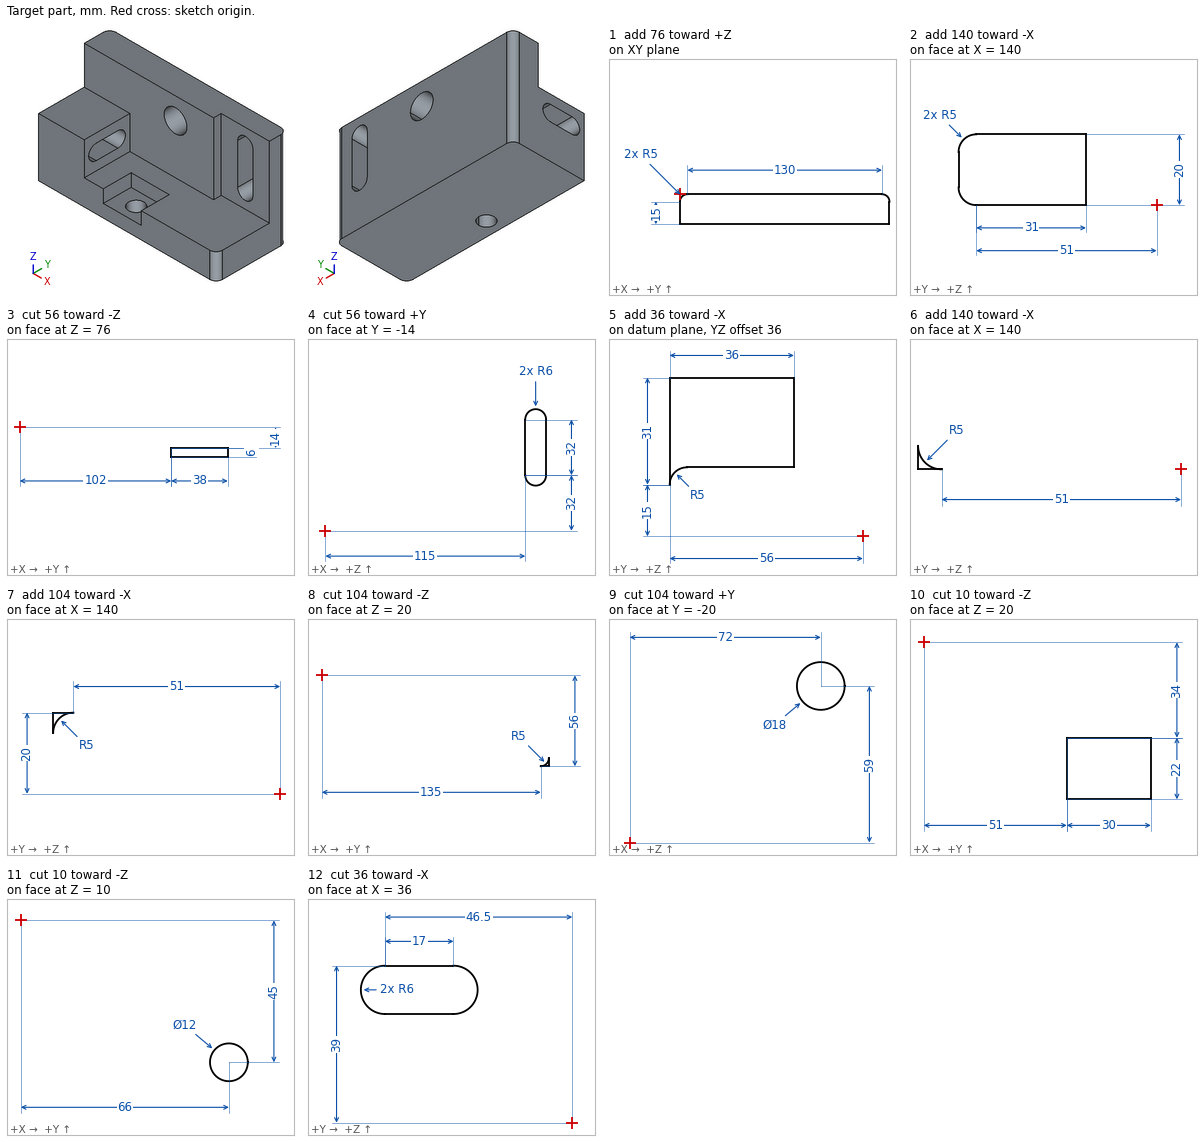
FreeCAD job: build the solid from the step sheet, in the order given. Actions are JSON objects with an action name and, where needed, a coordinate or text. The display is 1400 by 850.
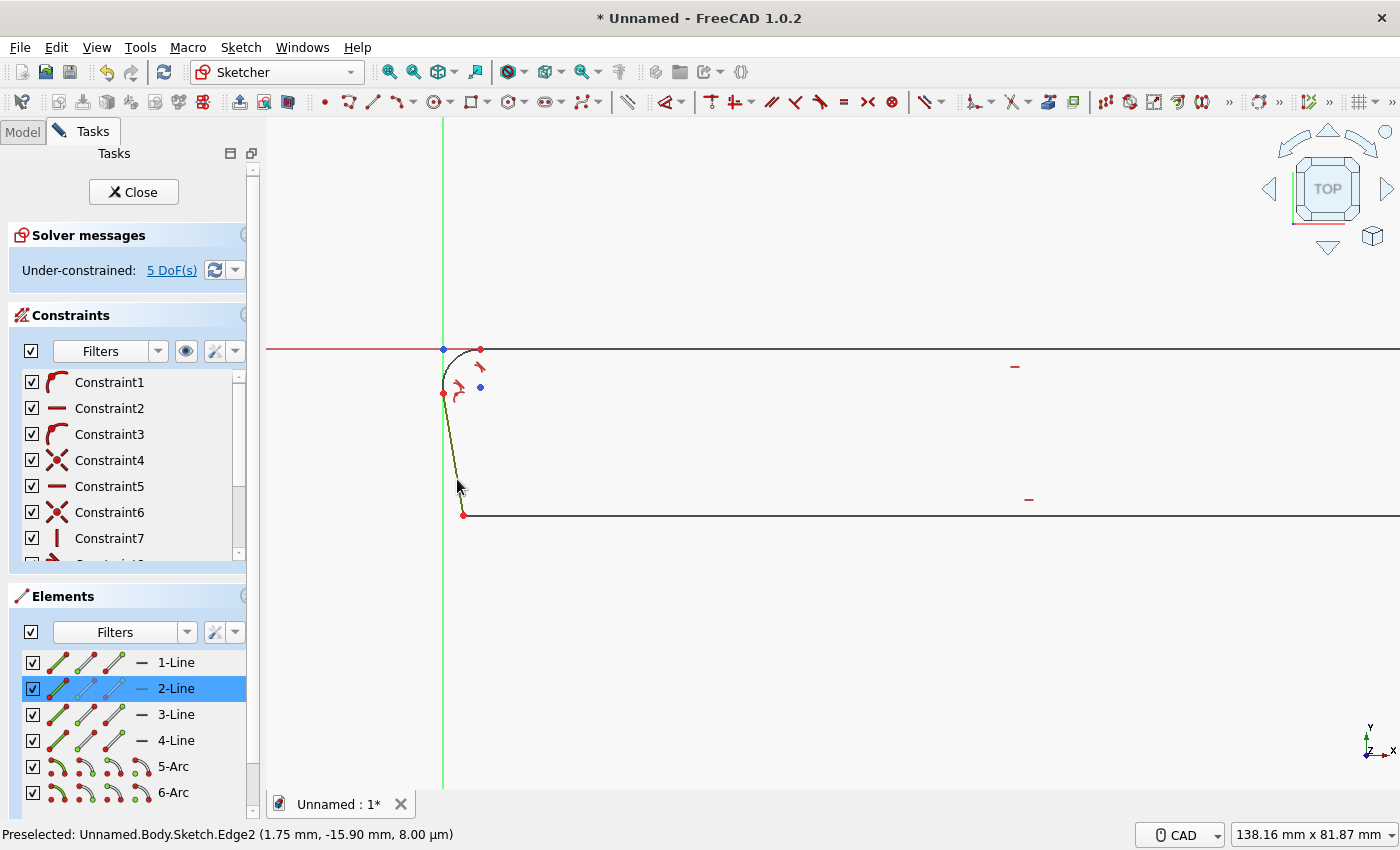
{"action": "key", "text": "v"}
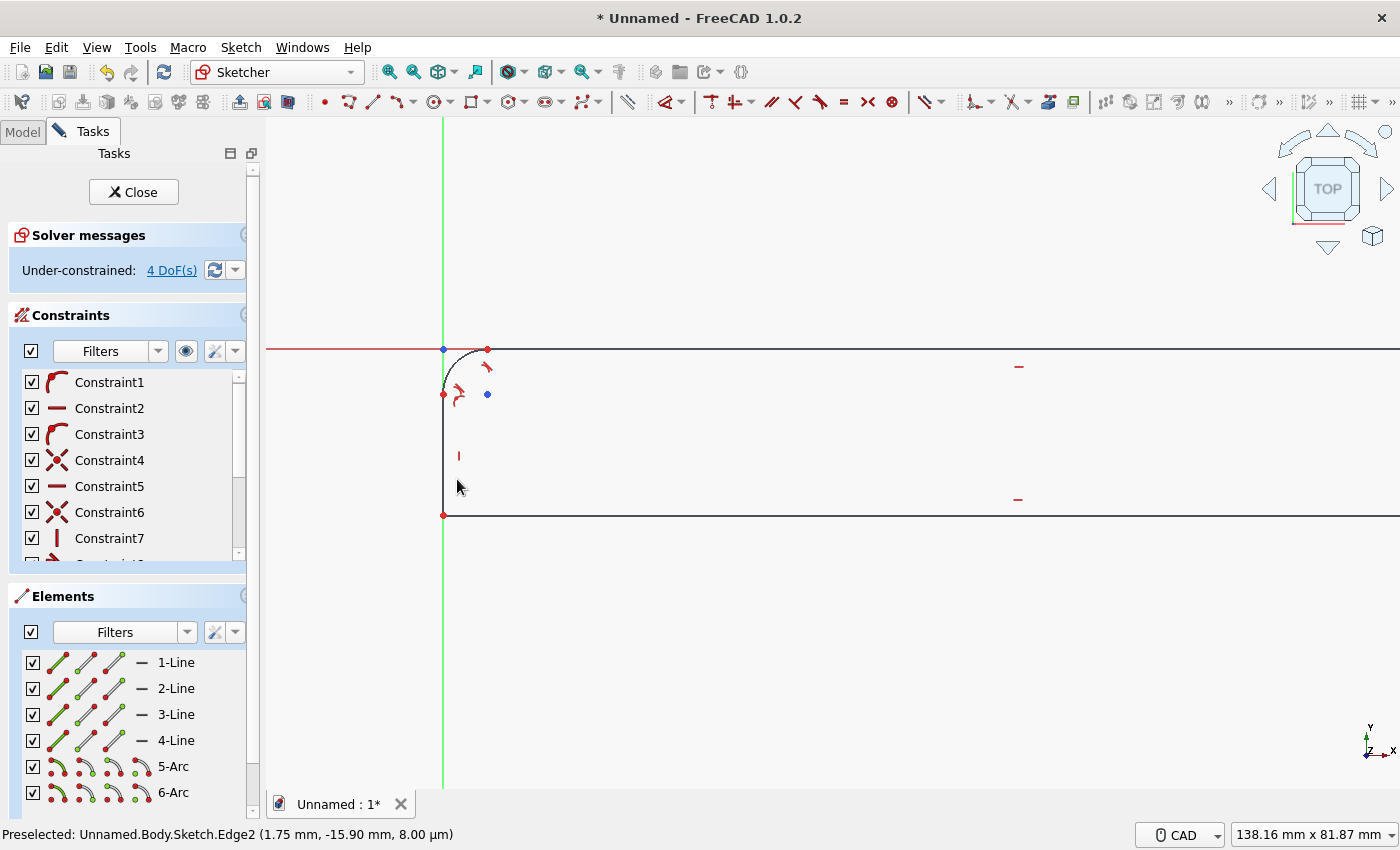
{"action": "left_click", "coordinate": [456, 362]}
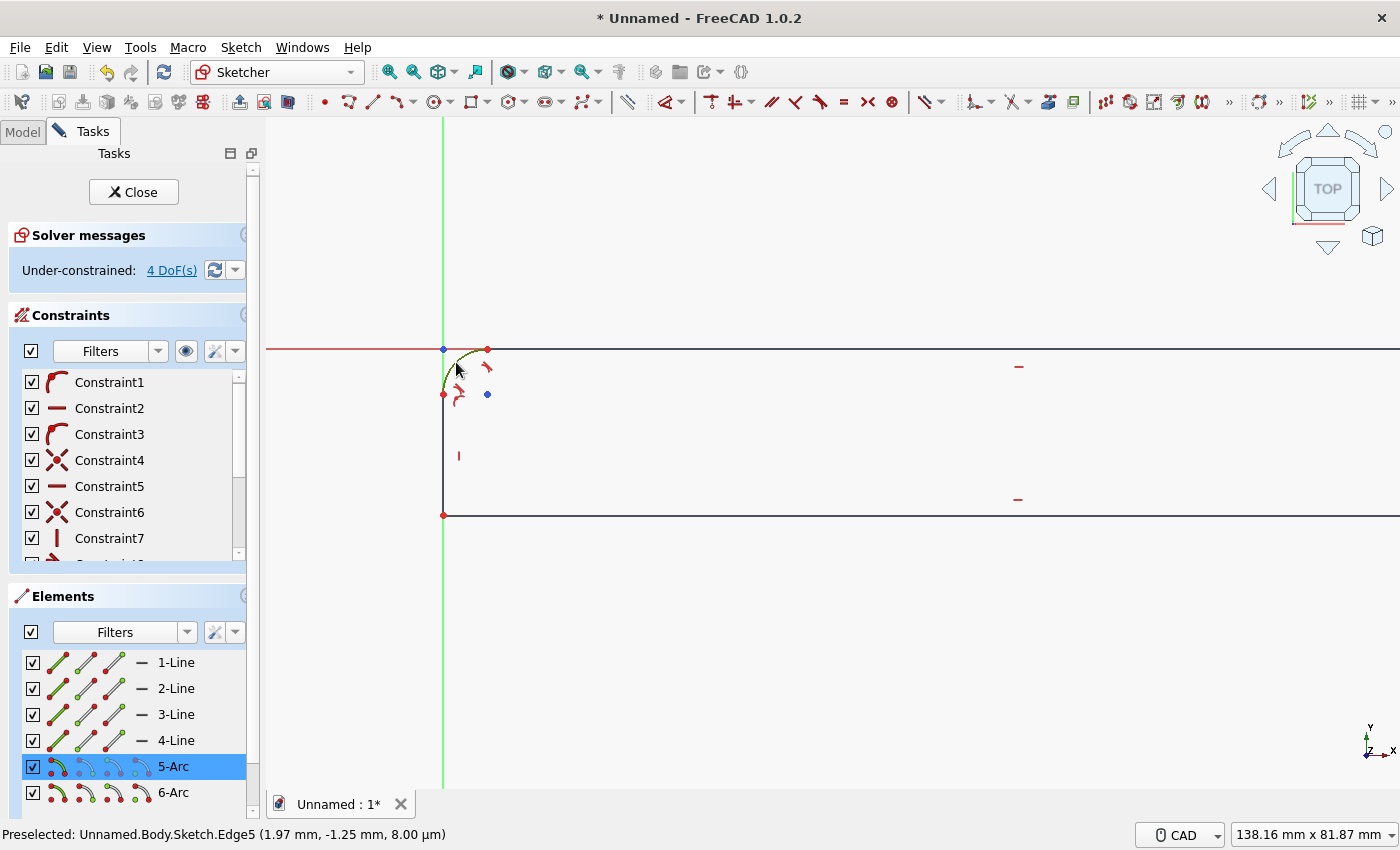
{"action": "scroll", "coordinate": [457, 479], "scroll_direction": "down", "scroll_amount": 3}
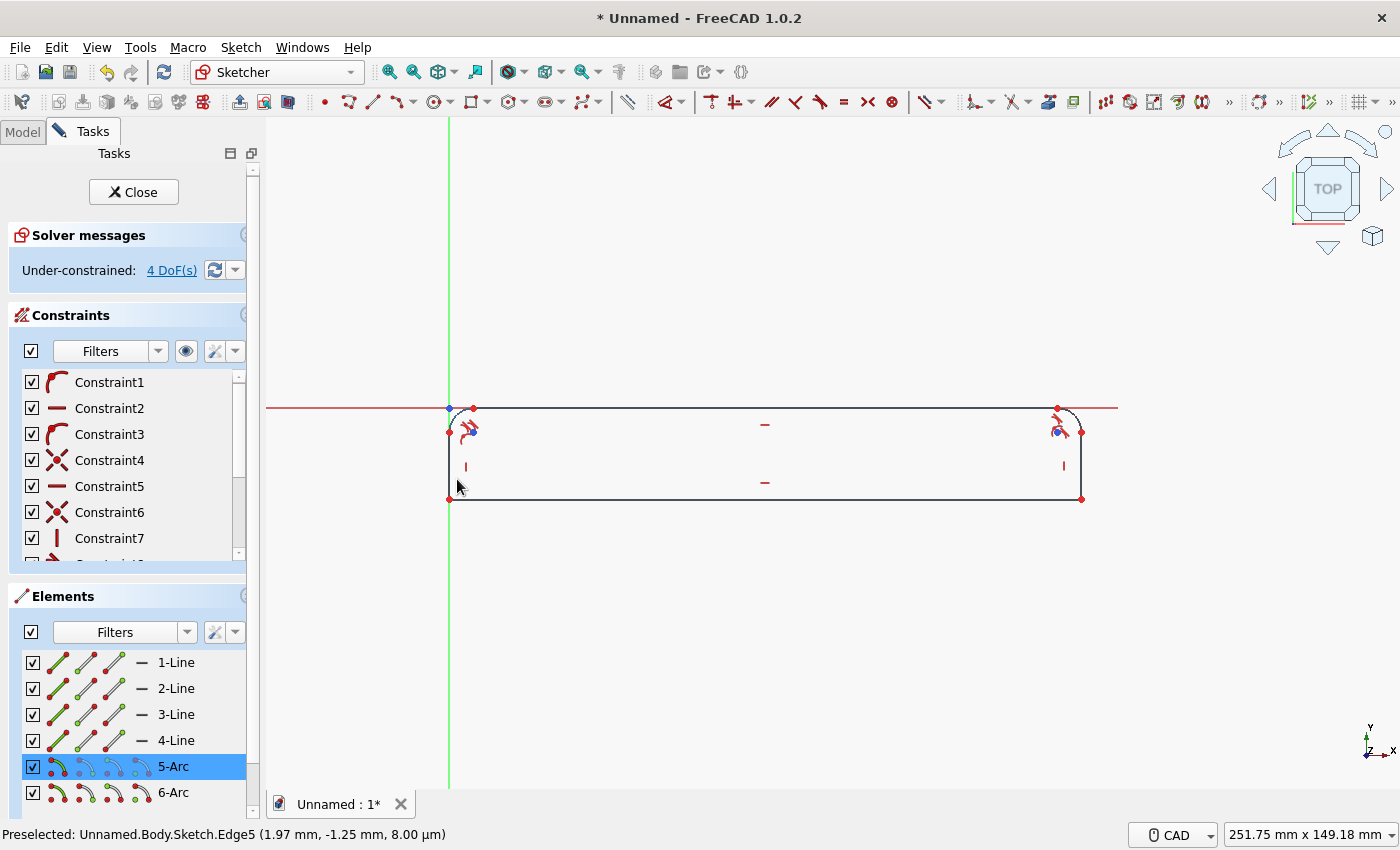
{"action": "scroll", "coordinate": [1079, 421], "scroll_direction": "up", "scroll_amount": 2}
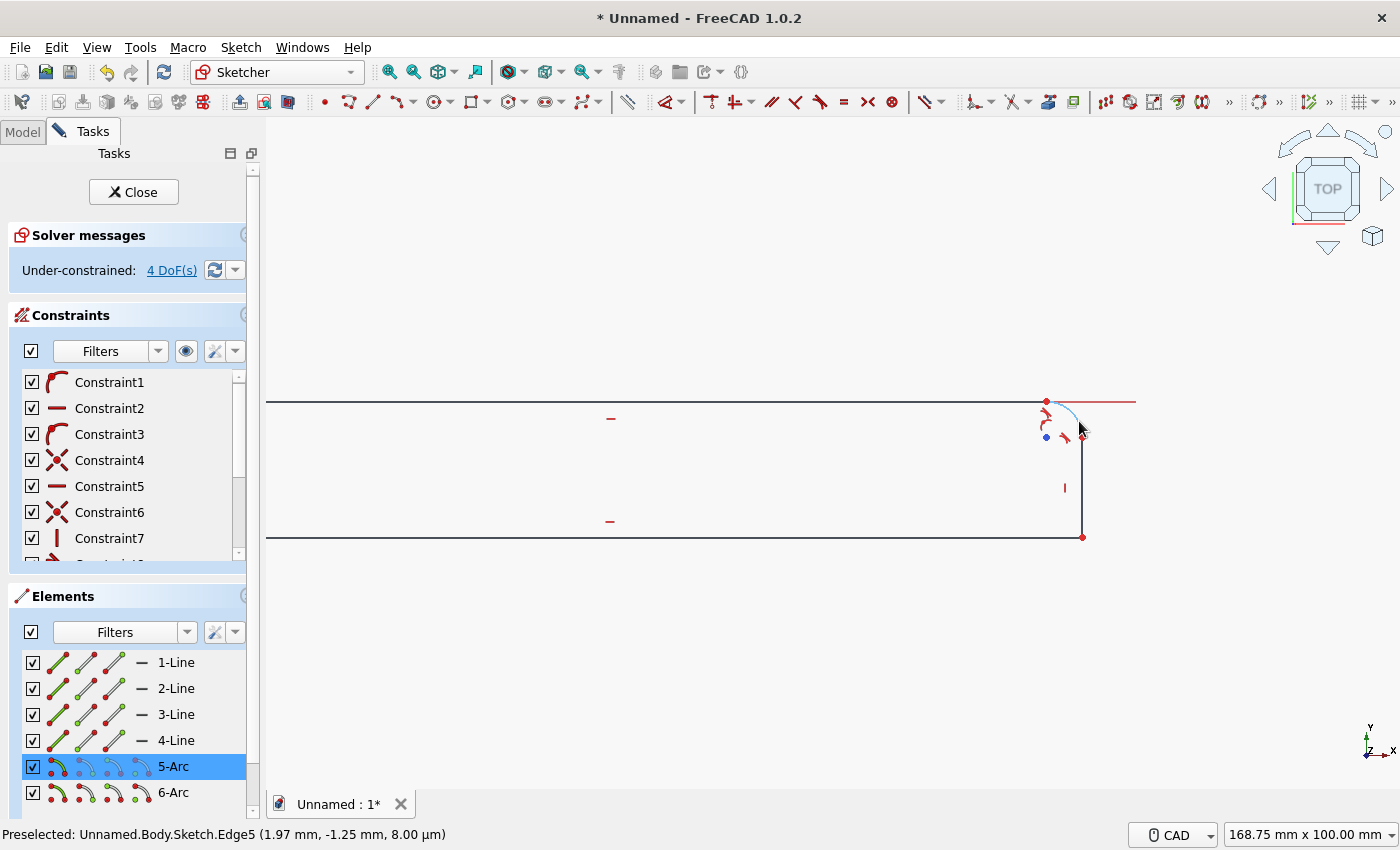
{"action": "left_click", "coordinate": [1078, 421]}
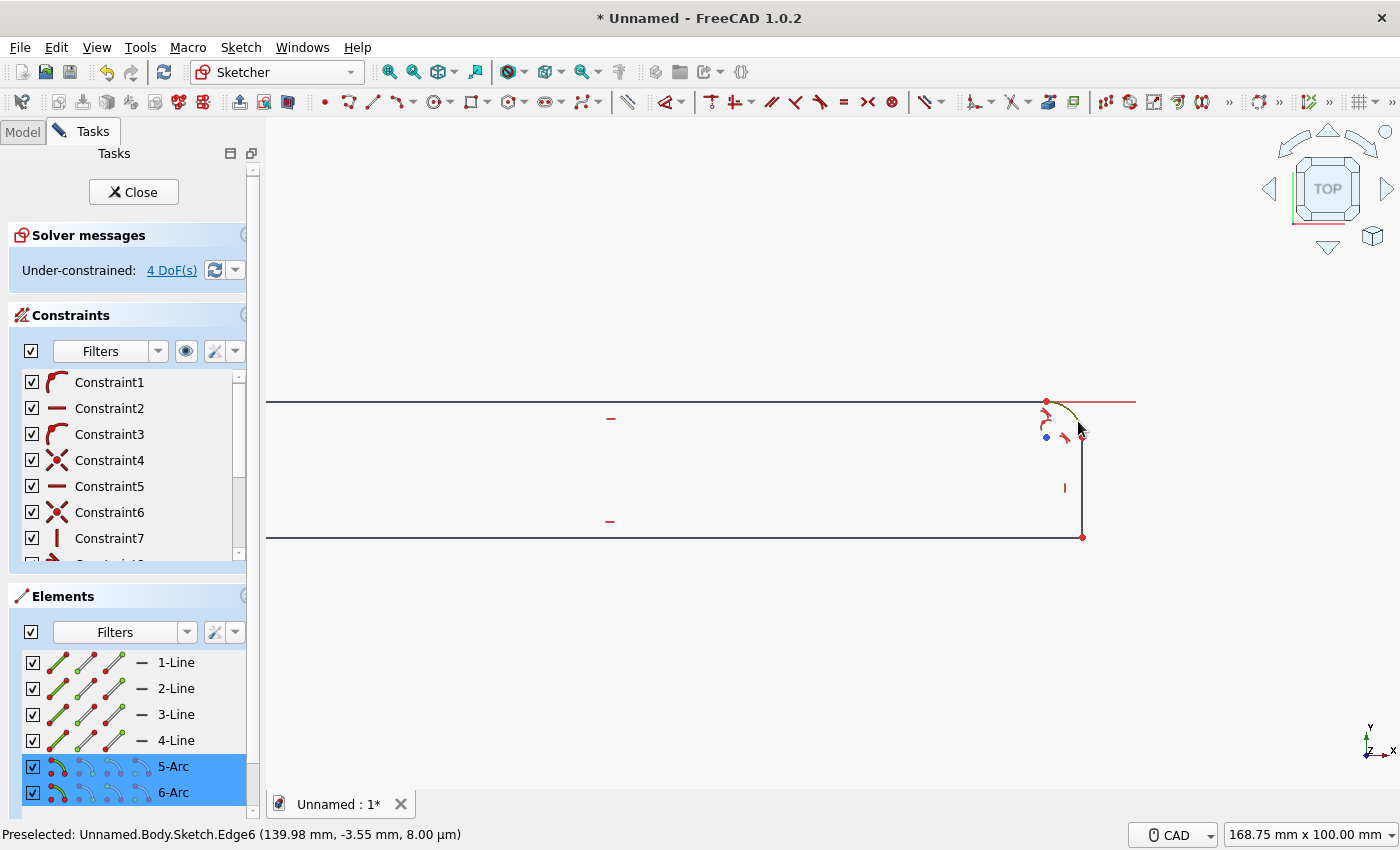
{"action": "left_click", "coordinate": [844, 102]}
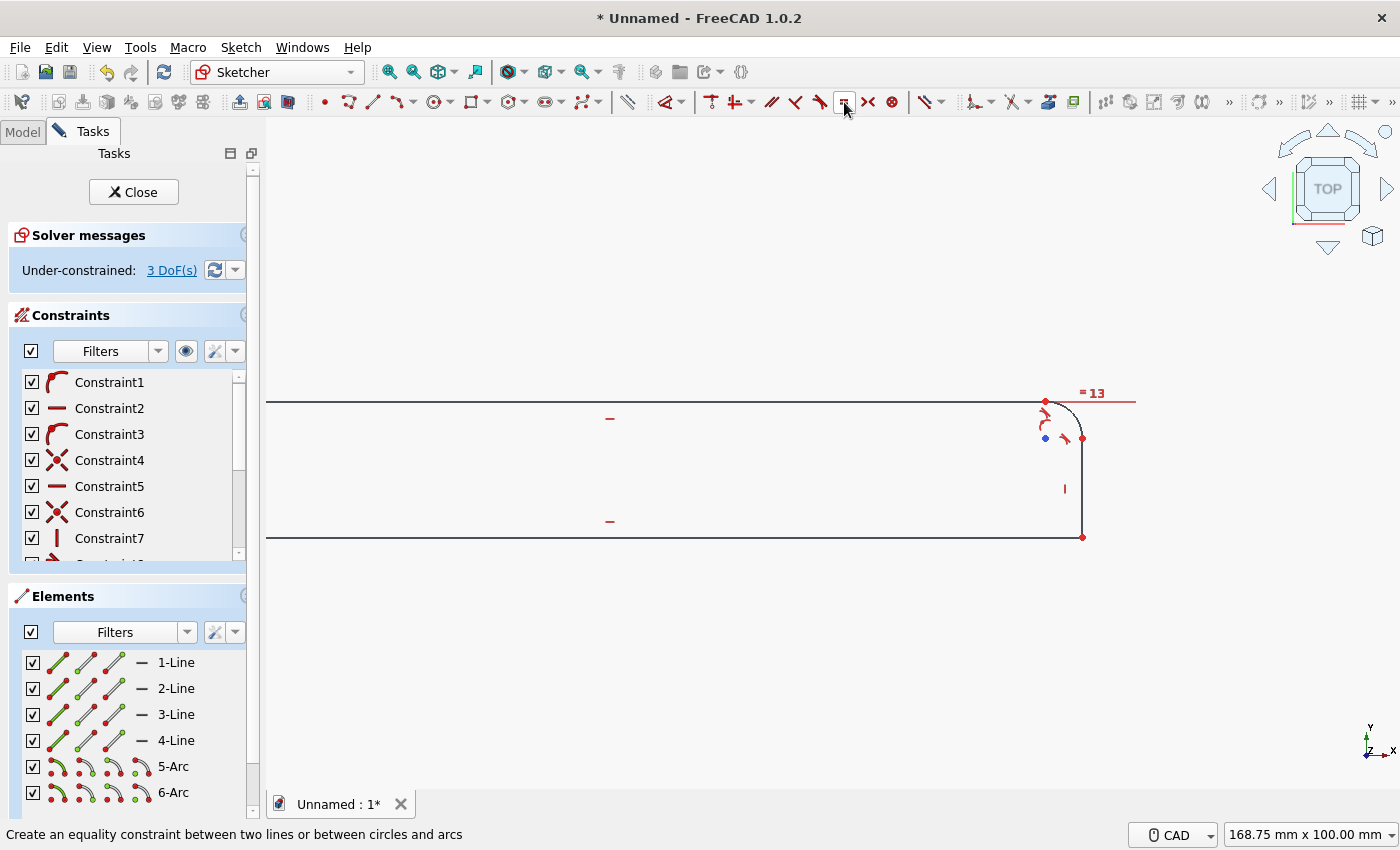
{"action": "left_click", "coordinate": [666, 102]}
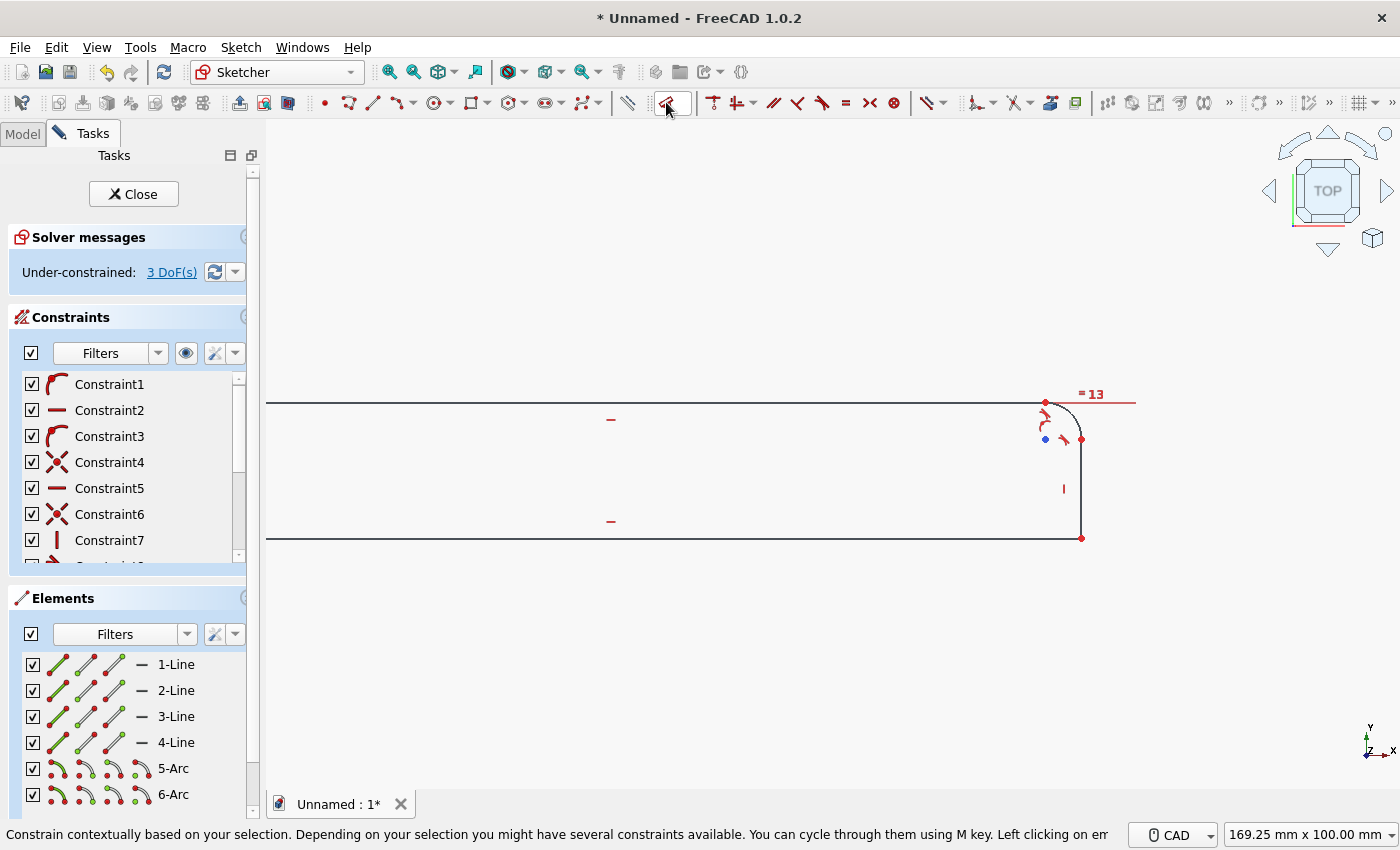
{"action": "scroll", "coordinate": [1078, 422], "scroll_direction": "down", "scroll_amount": 2}